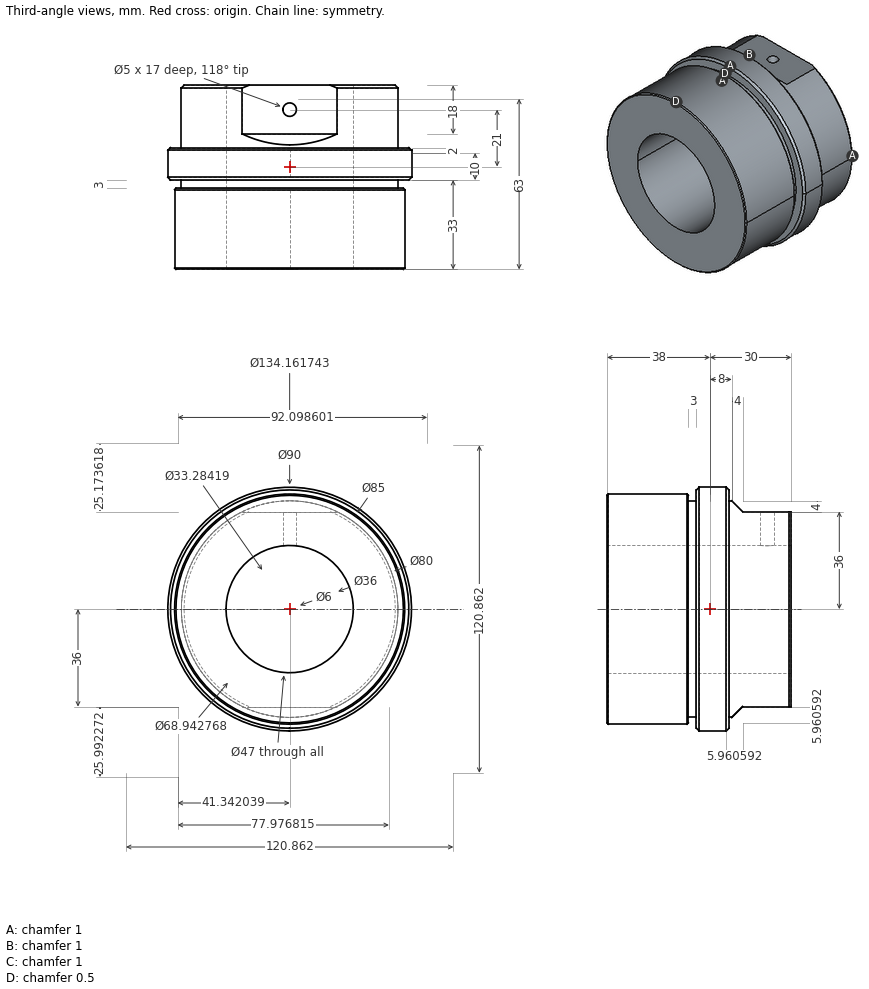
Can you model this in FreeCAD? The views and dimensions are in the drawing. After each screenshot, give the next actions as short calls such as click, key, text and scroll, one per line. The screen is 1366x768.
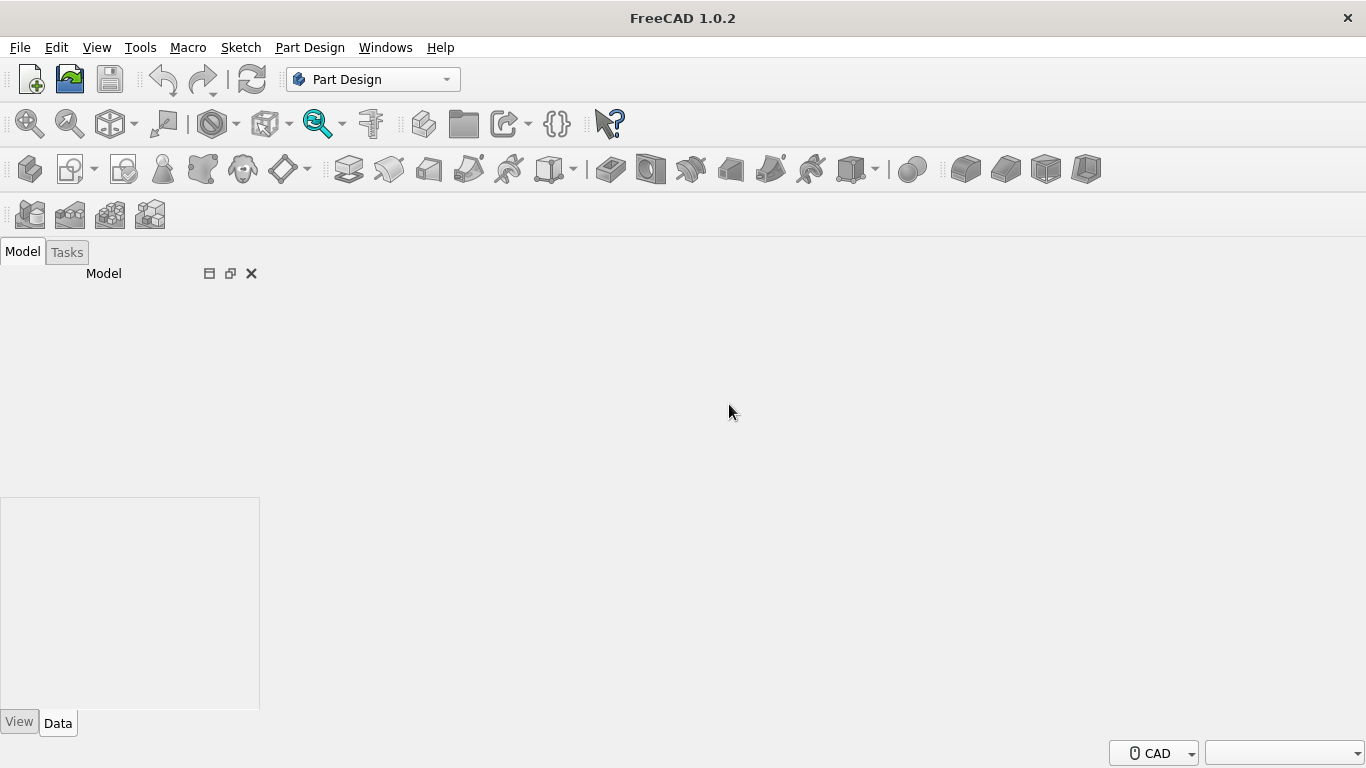
click(30, 80)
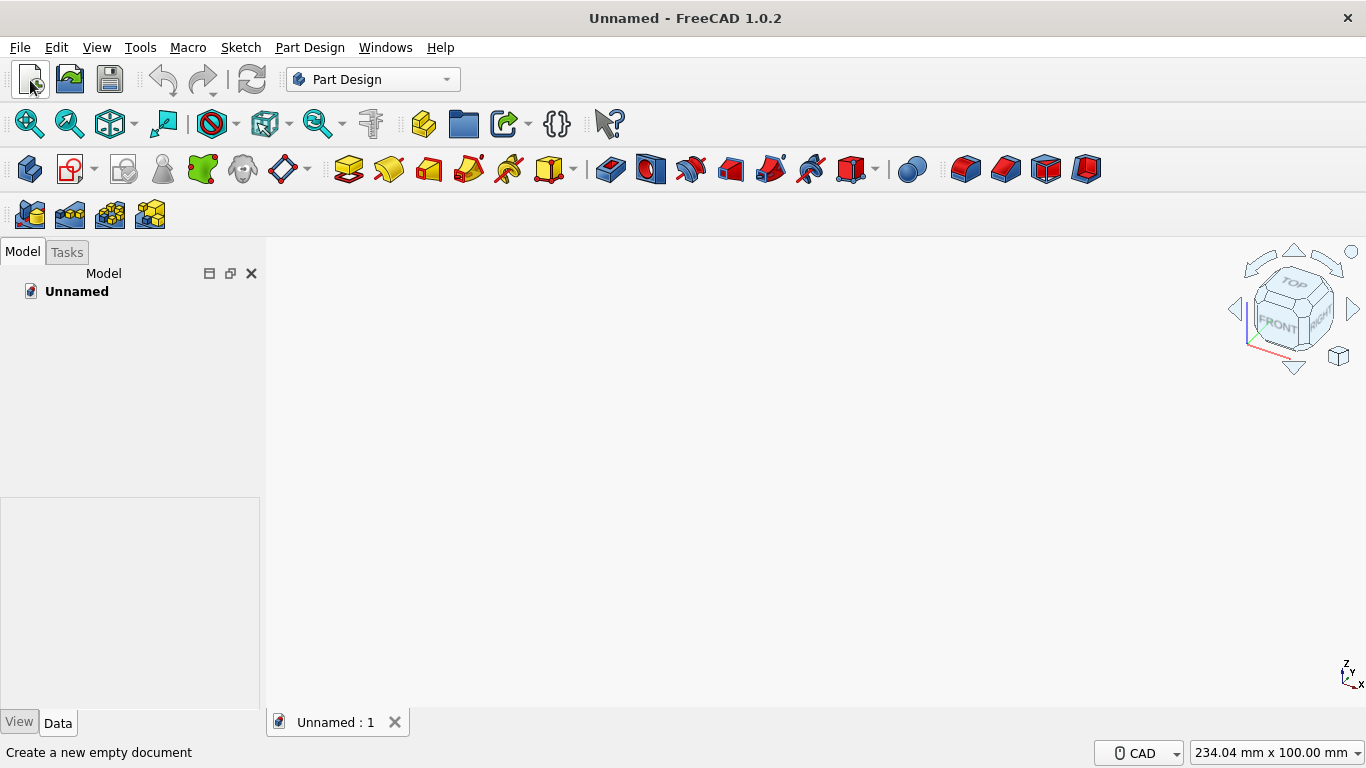
click(70, 170)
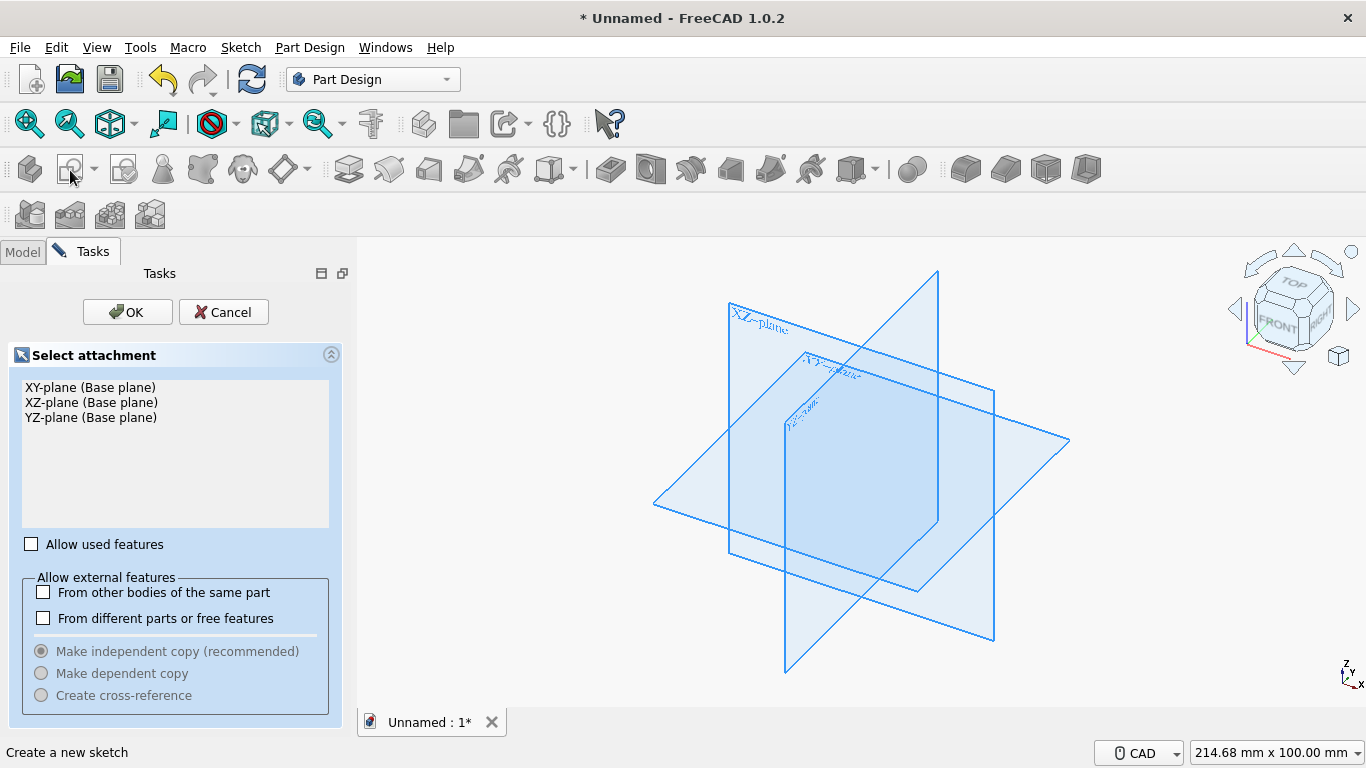
click(82, 402)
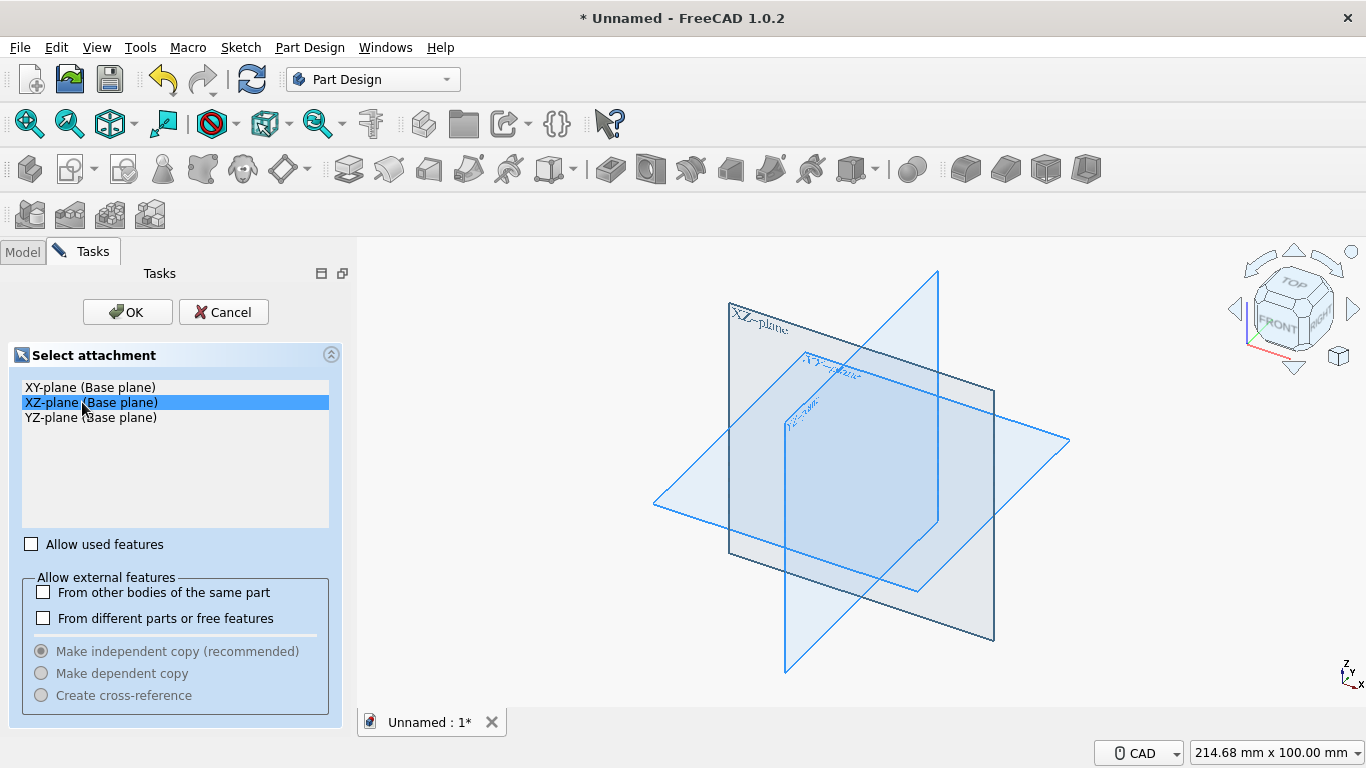
click(128, 312)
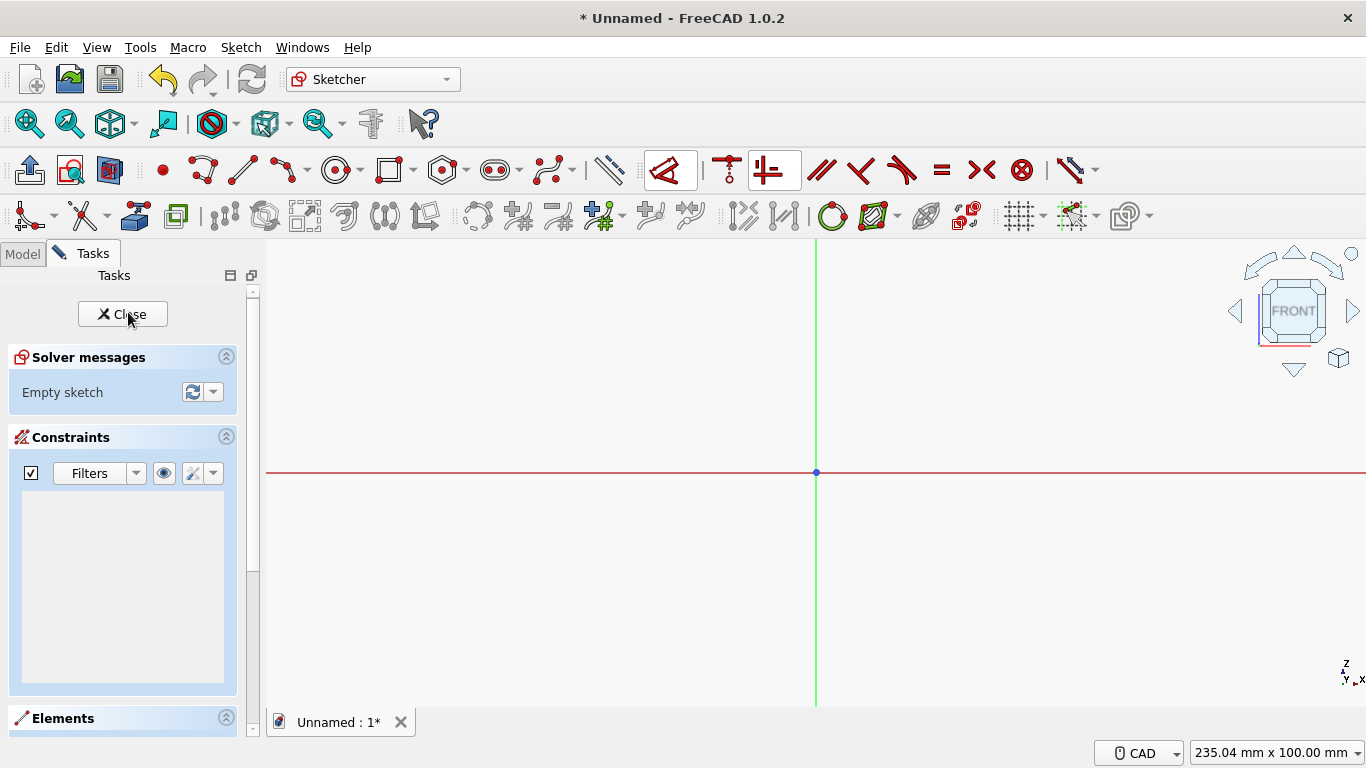
scroll(438, 473, down, 1)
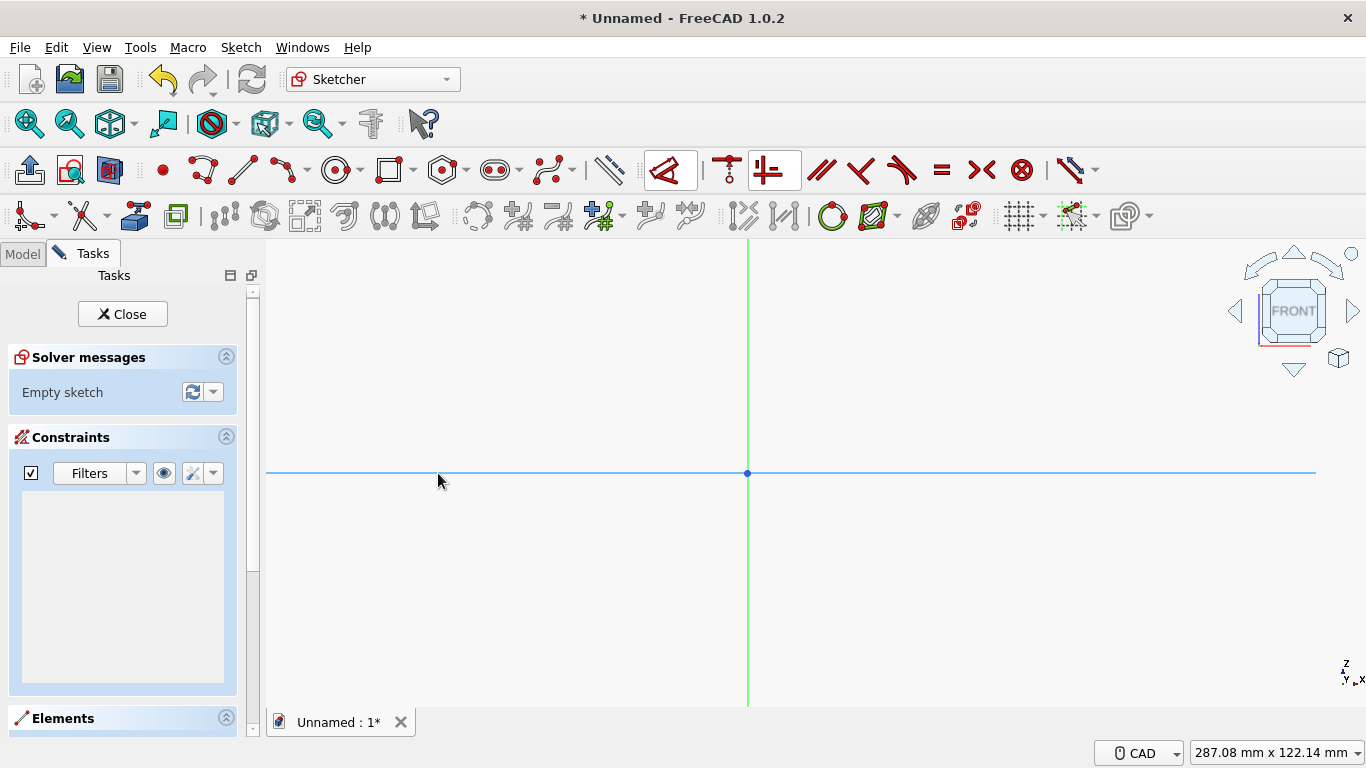
click(336, 170)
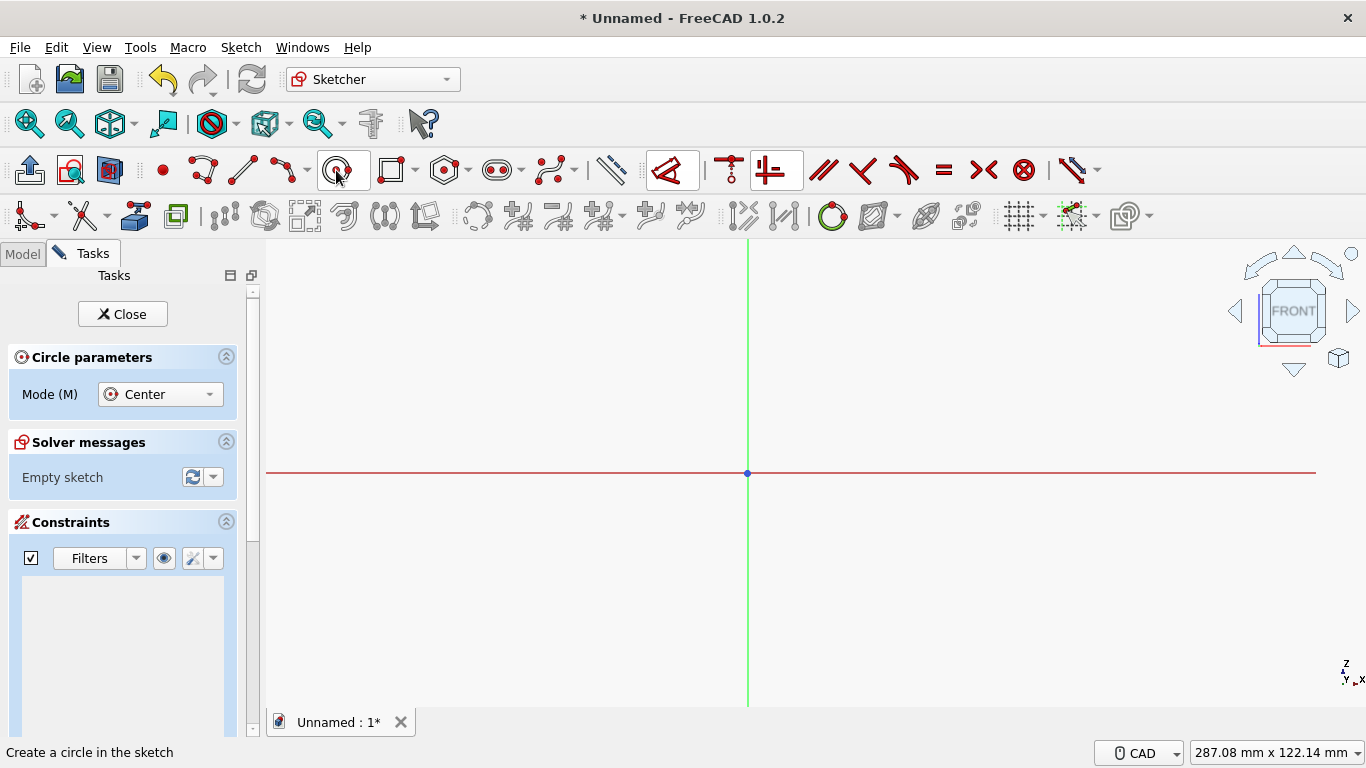
click(748, 473)
click(856, 365)
key(Escape)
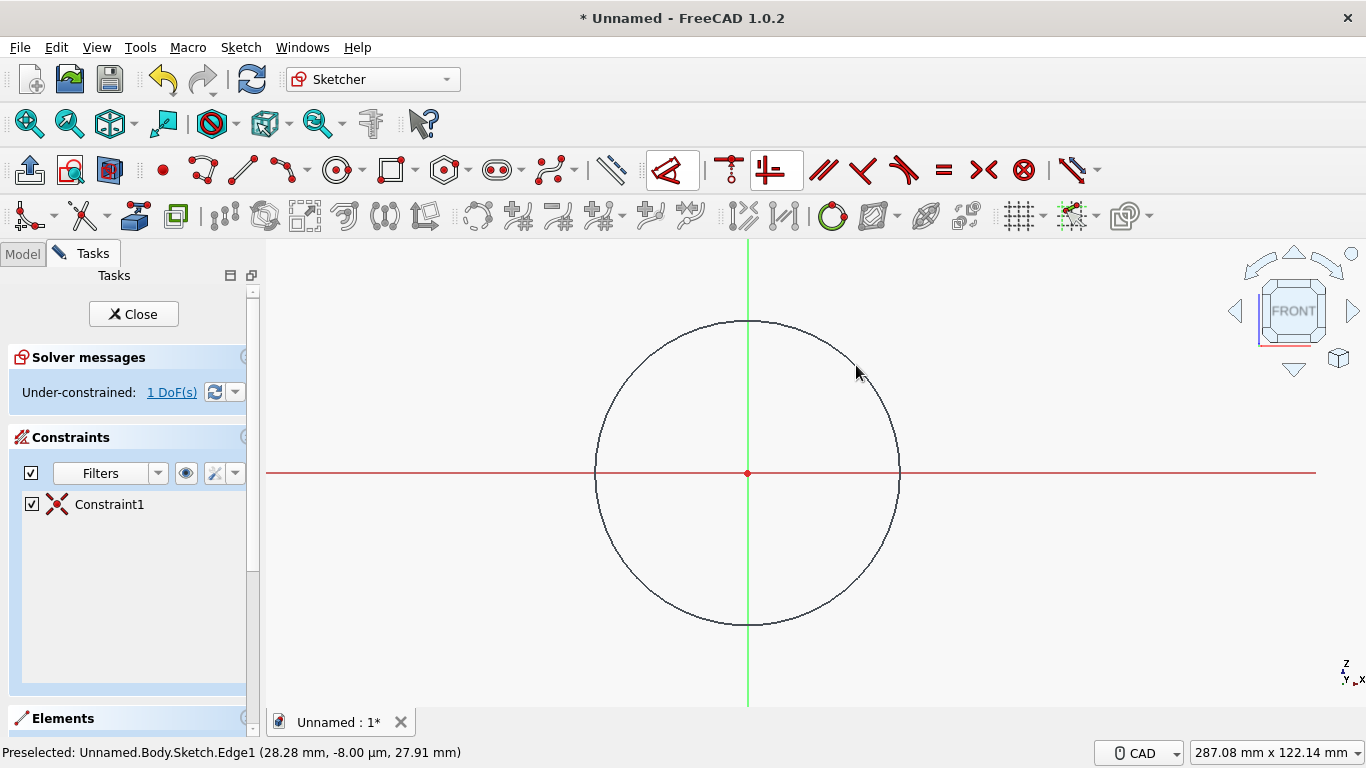
click(666, 170)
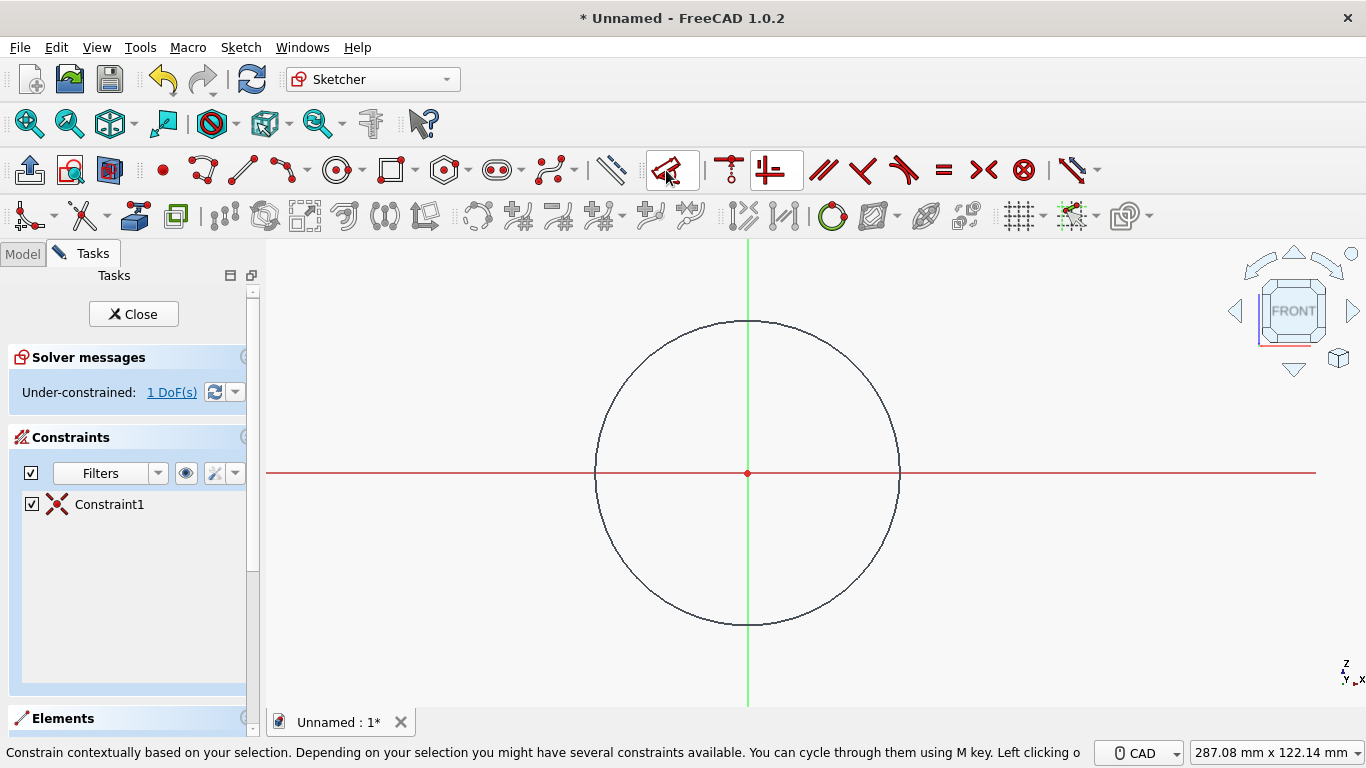
click(855, 365)
click(878, 342)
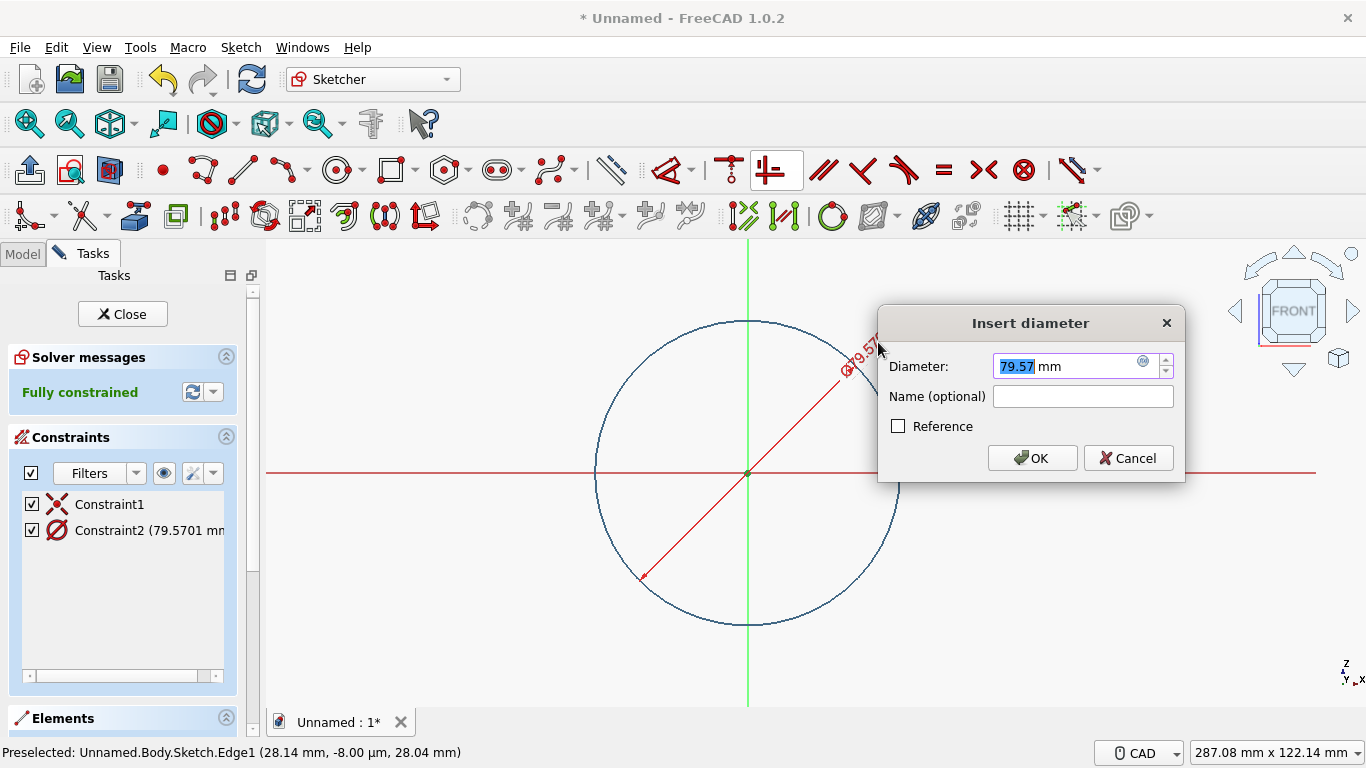
text(80)
key(Return)
key(Escape)